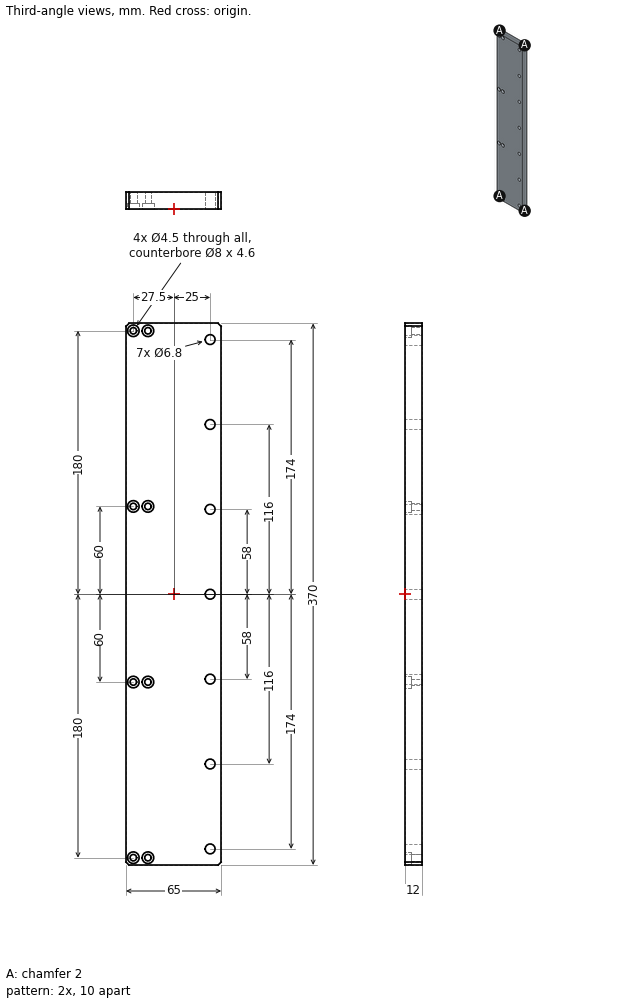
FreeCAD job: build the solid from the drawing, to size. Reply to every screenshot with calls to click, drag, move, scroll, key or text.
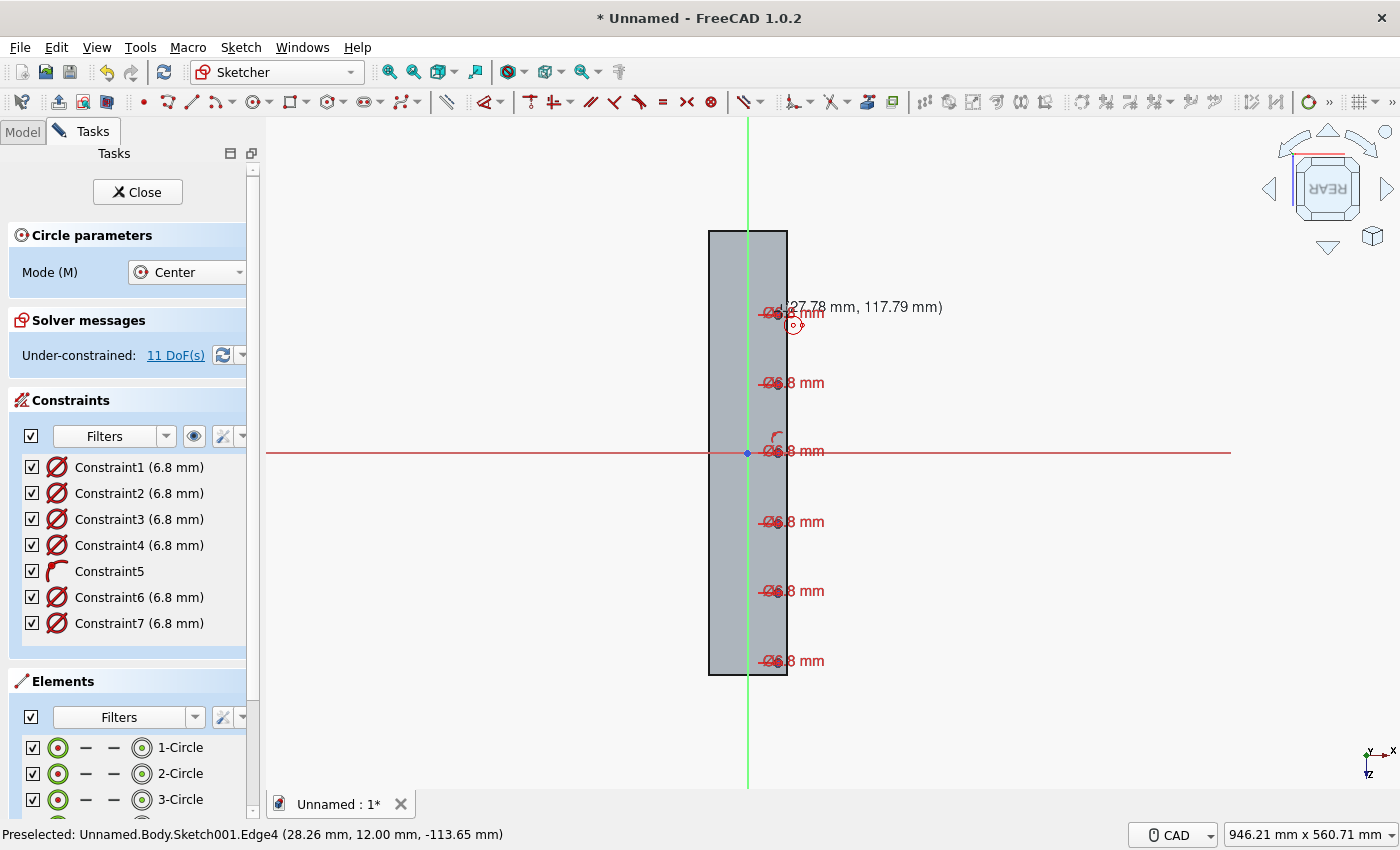
scroll(778, 245, up, 9)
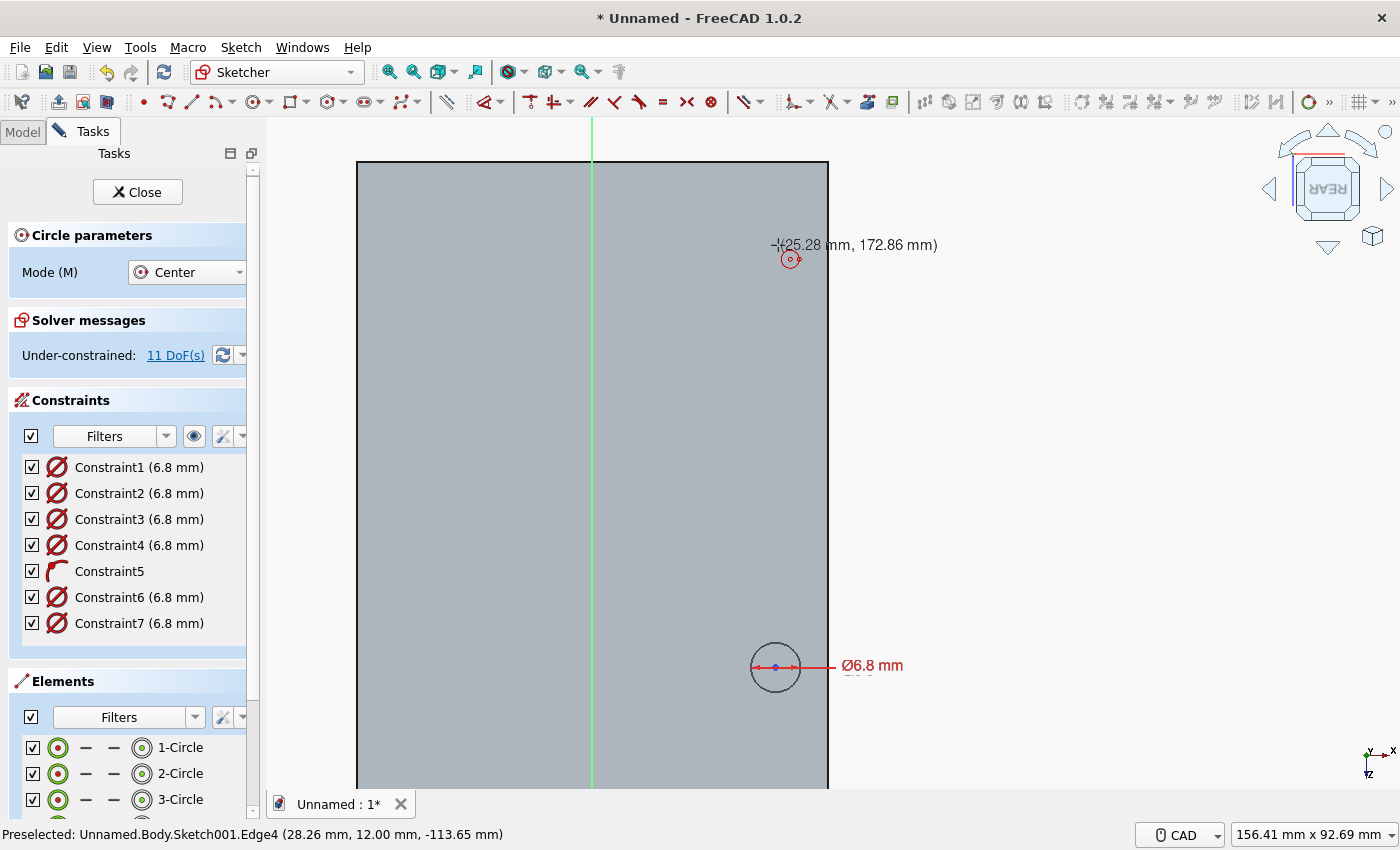
scroll(778, 245, down, 9)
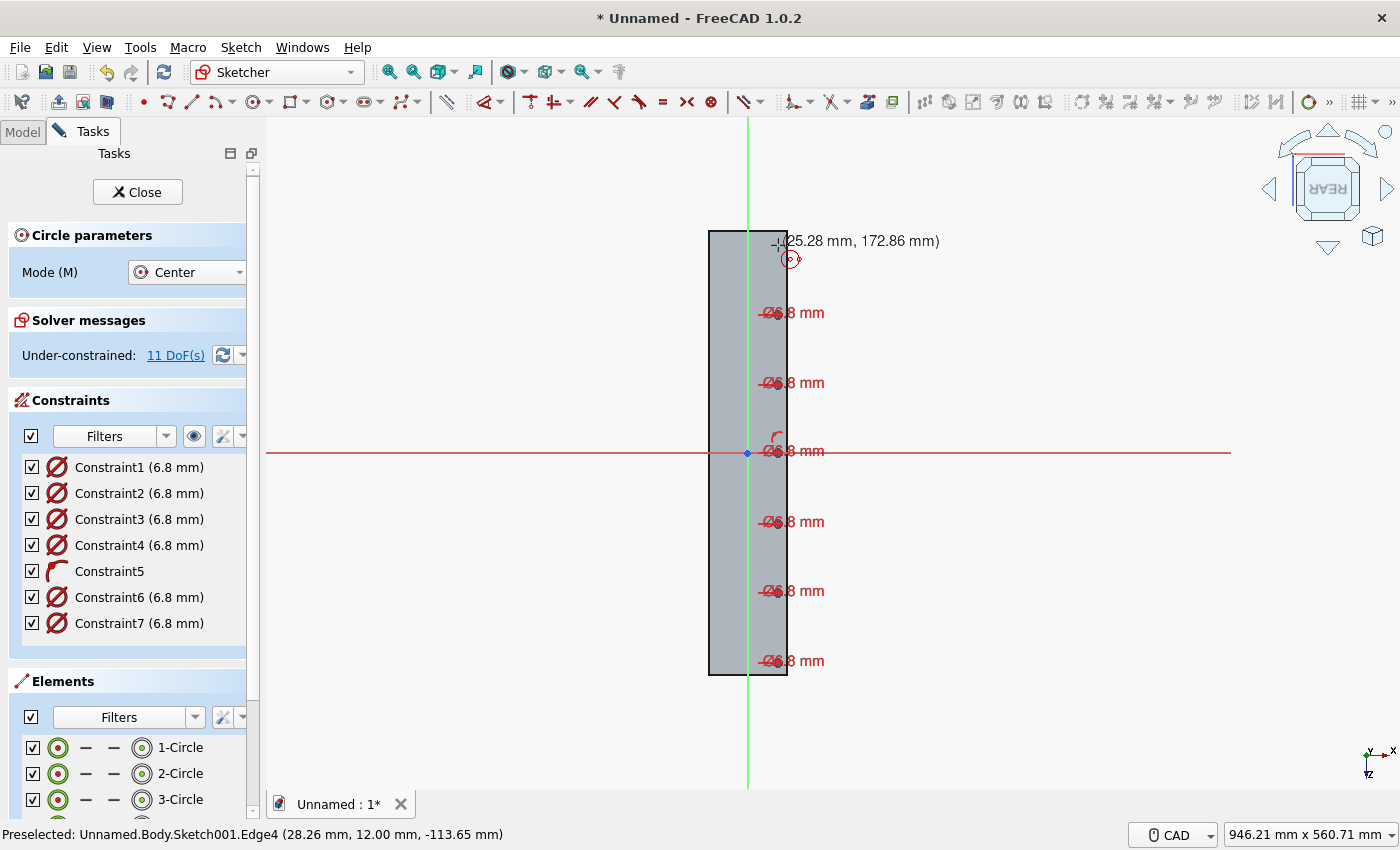
click(778, 245)
move(781, 242)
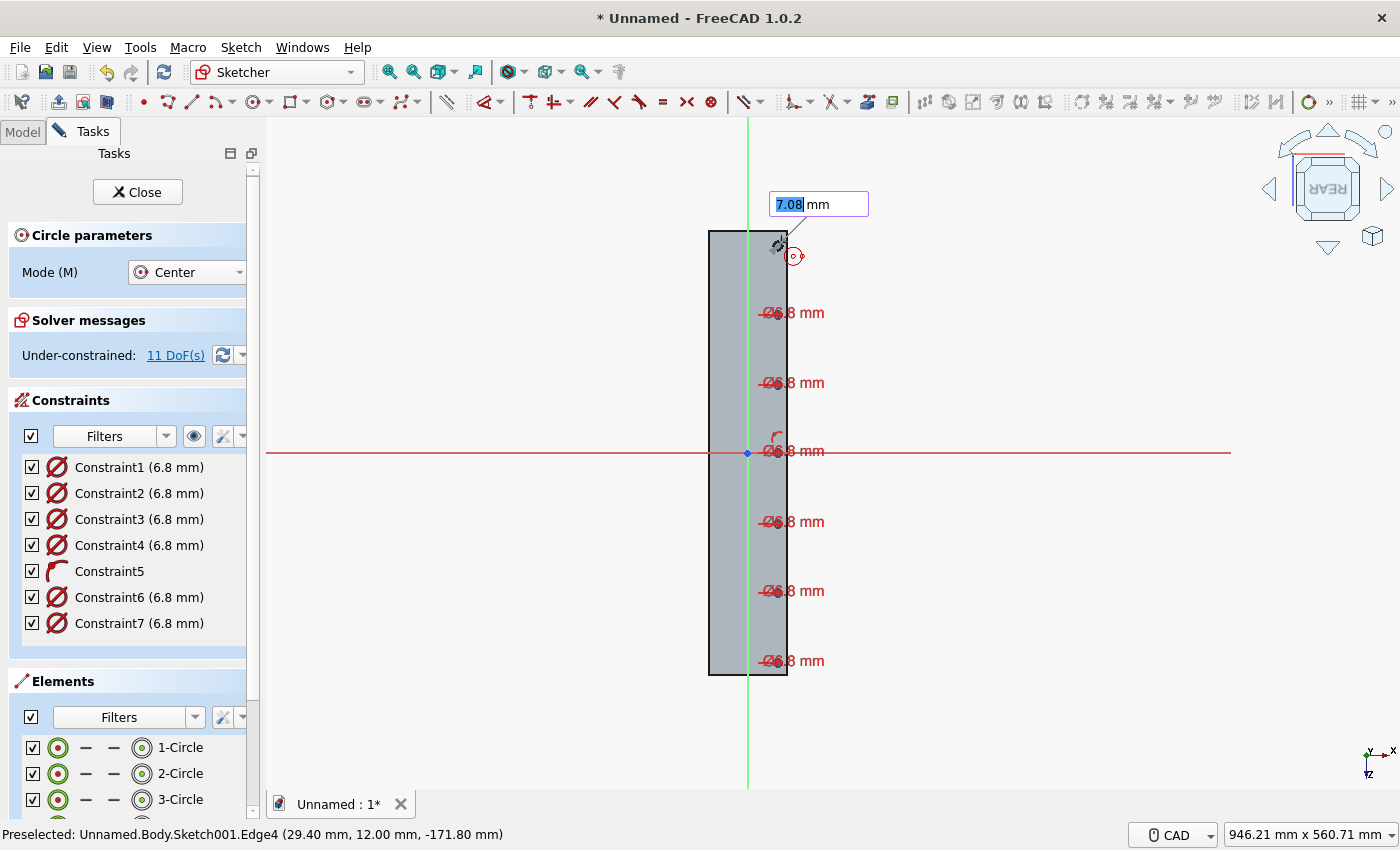
text(6.8)
key(Return)
key(Escape)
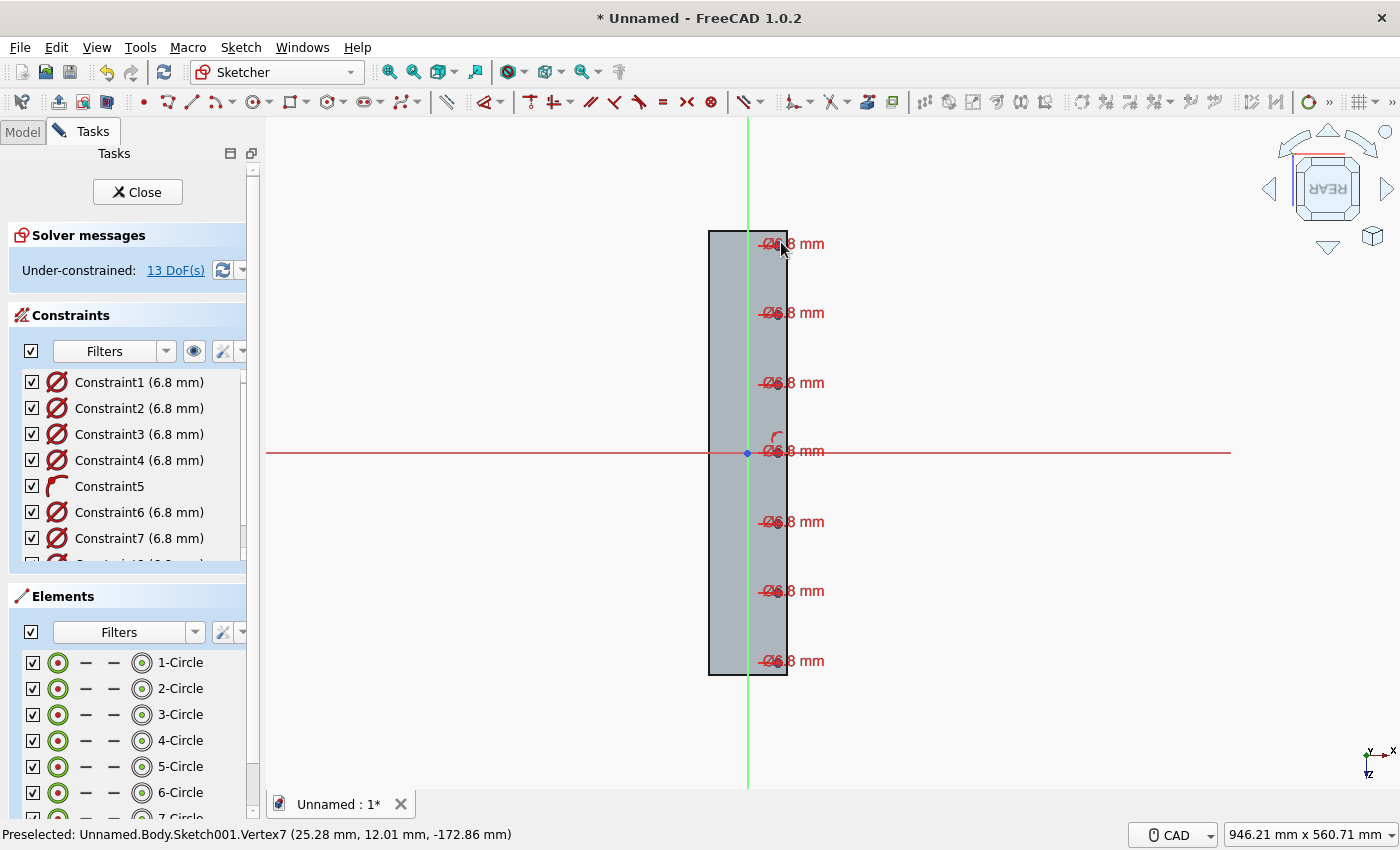
click(778, 663)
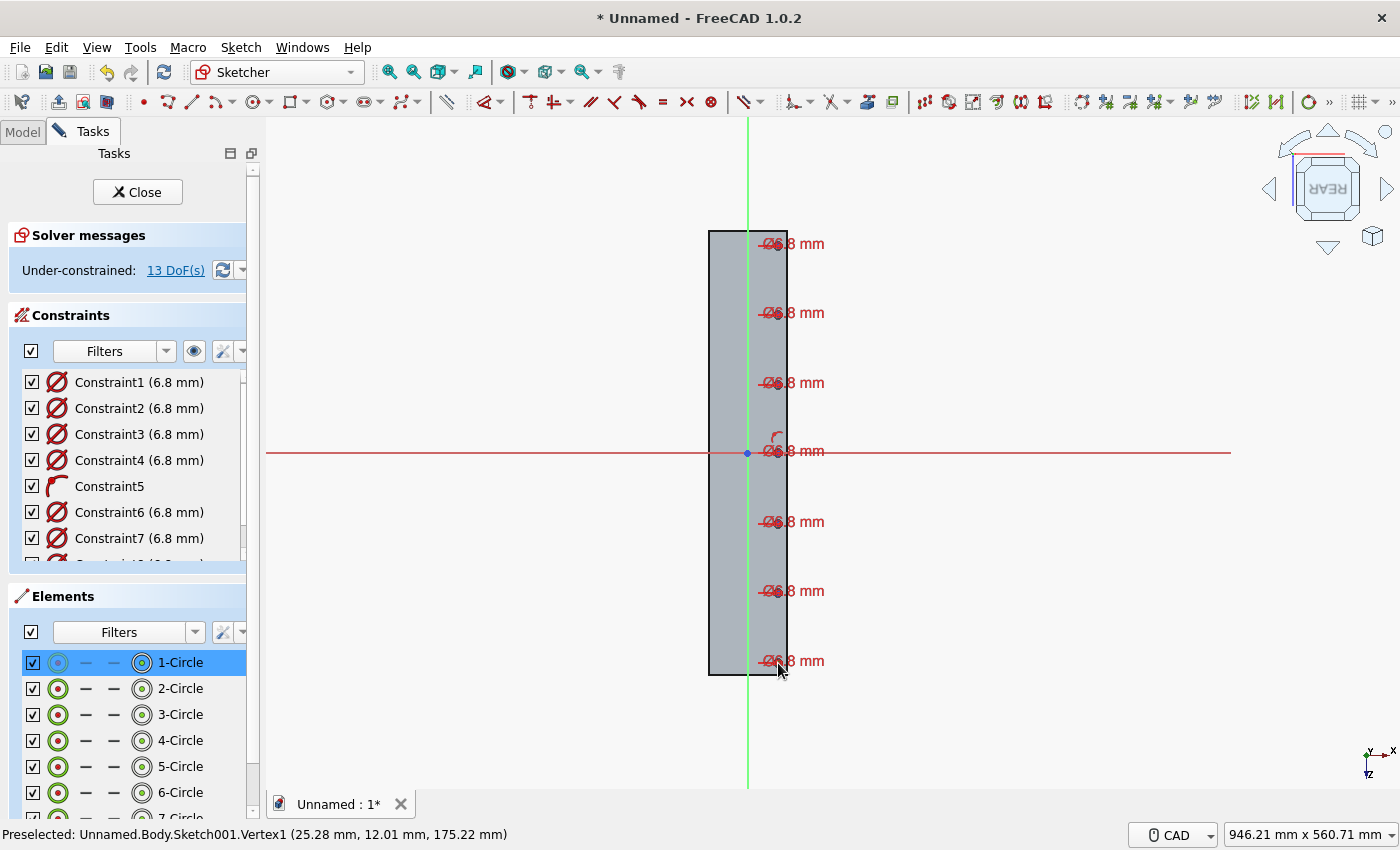
click(778, 593)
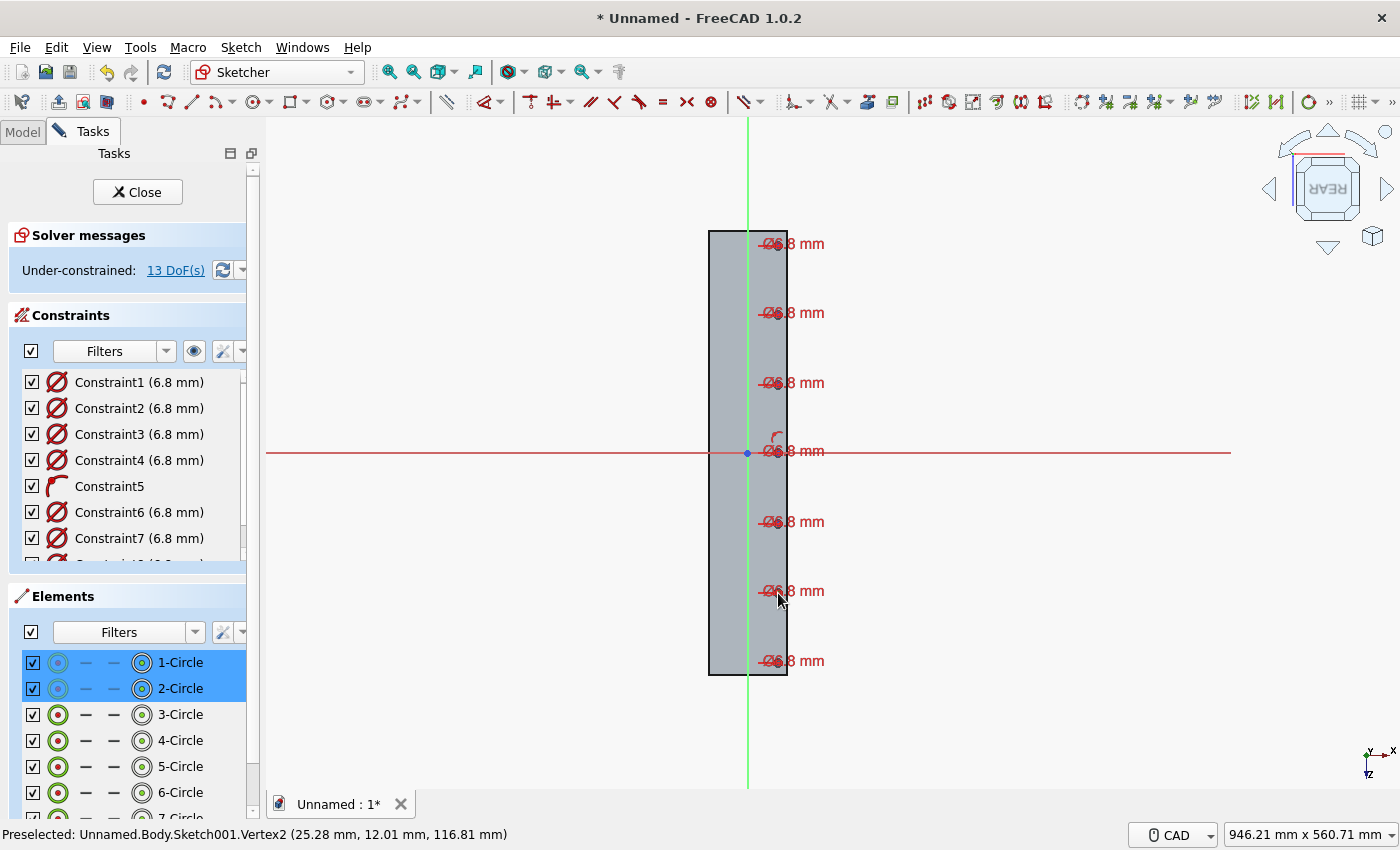
key(v)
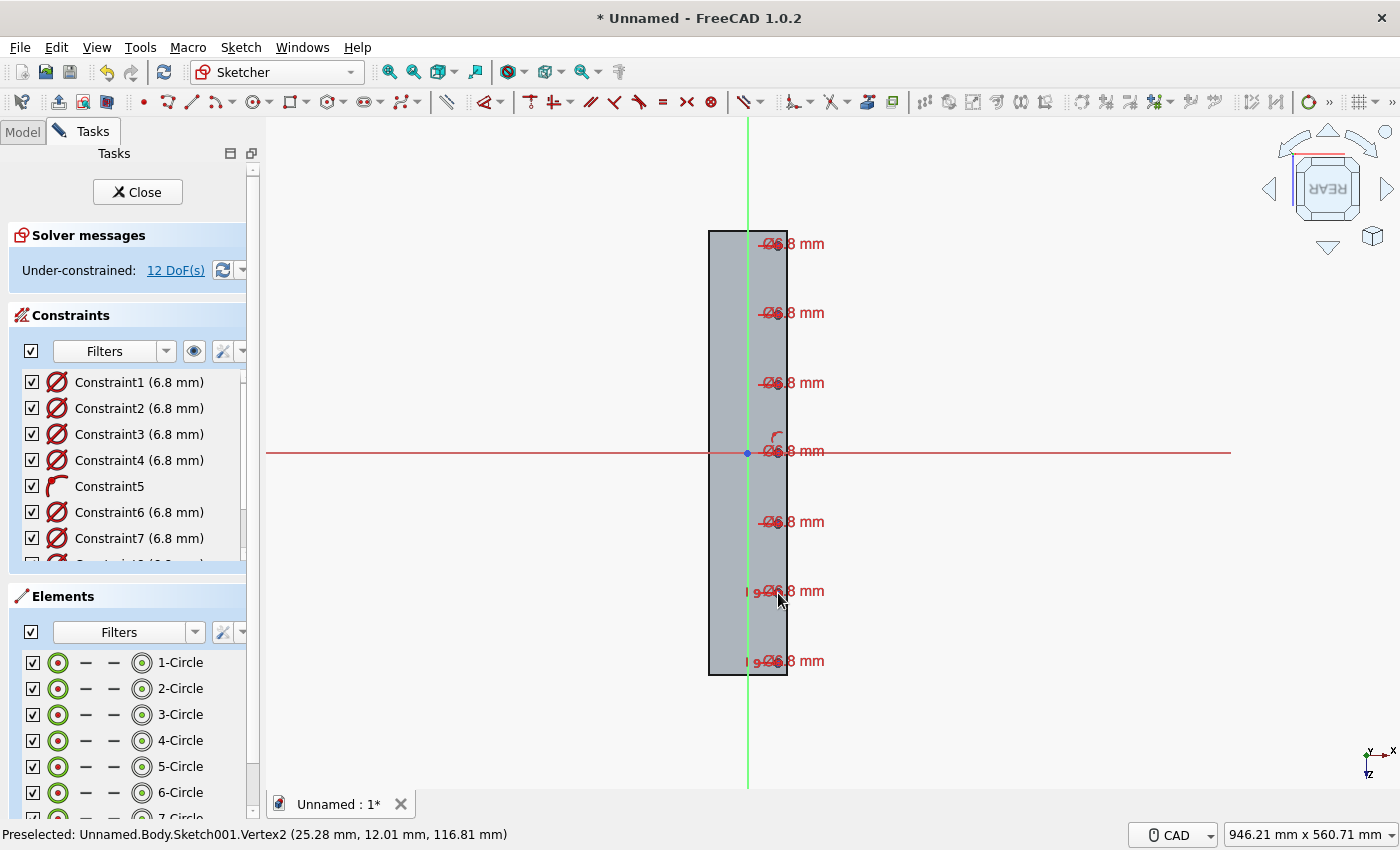
click(778, 593)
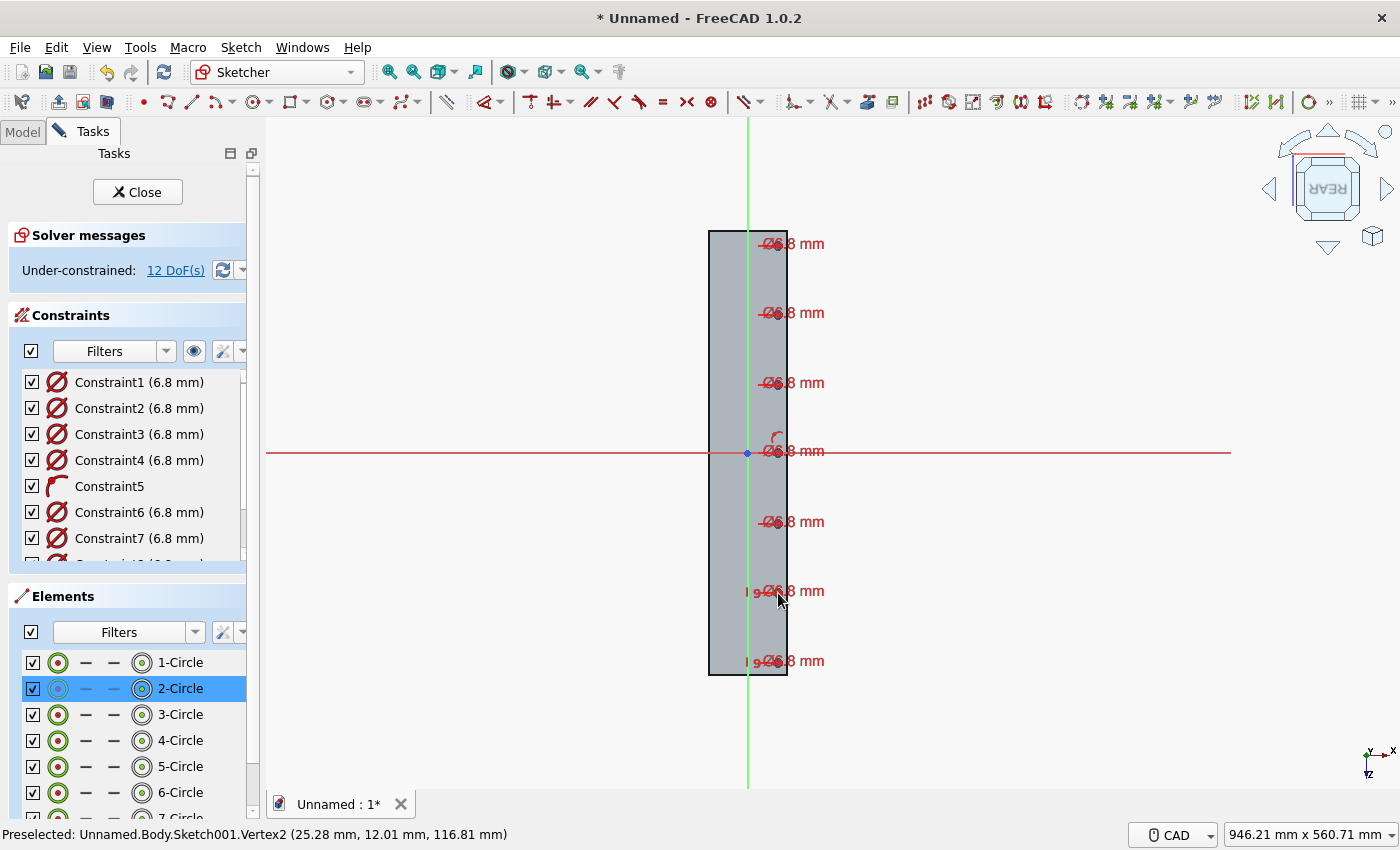
click(778, 524)